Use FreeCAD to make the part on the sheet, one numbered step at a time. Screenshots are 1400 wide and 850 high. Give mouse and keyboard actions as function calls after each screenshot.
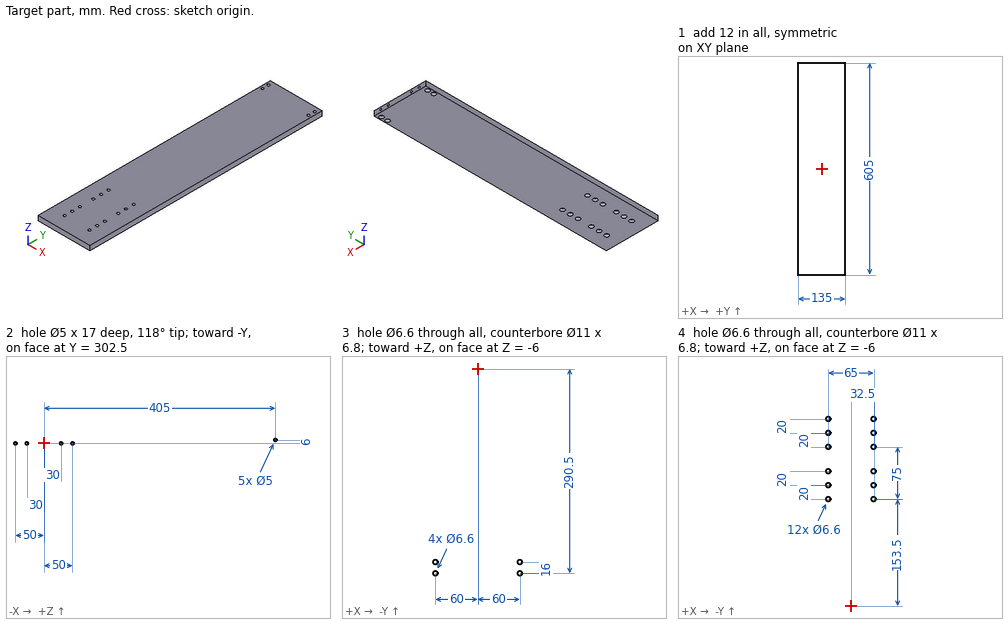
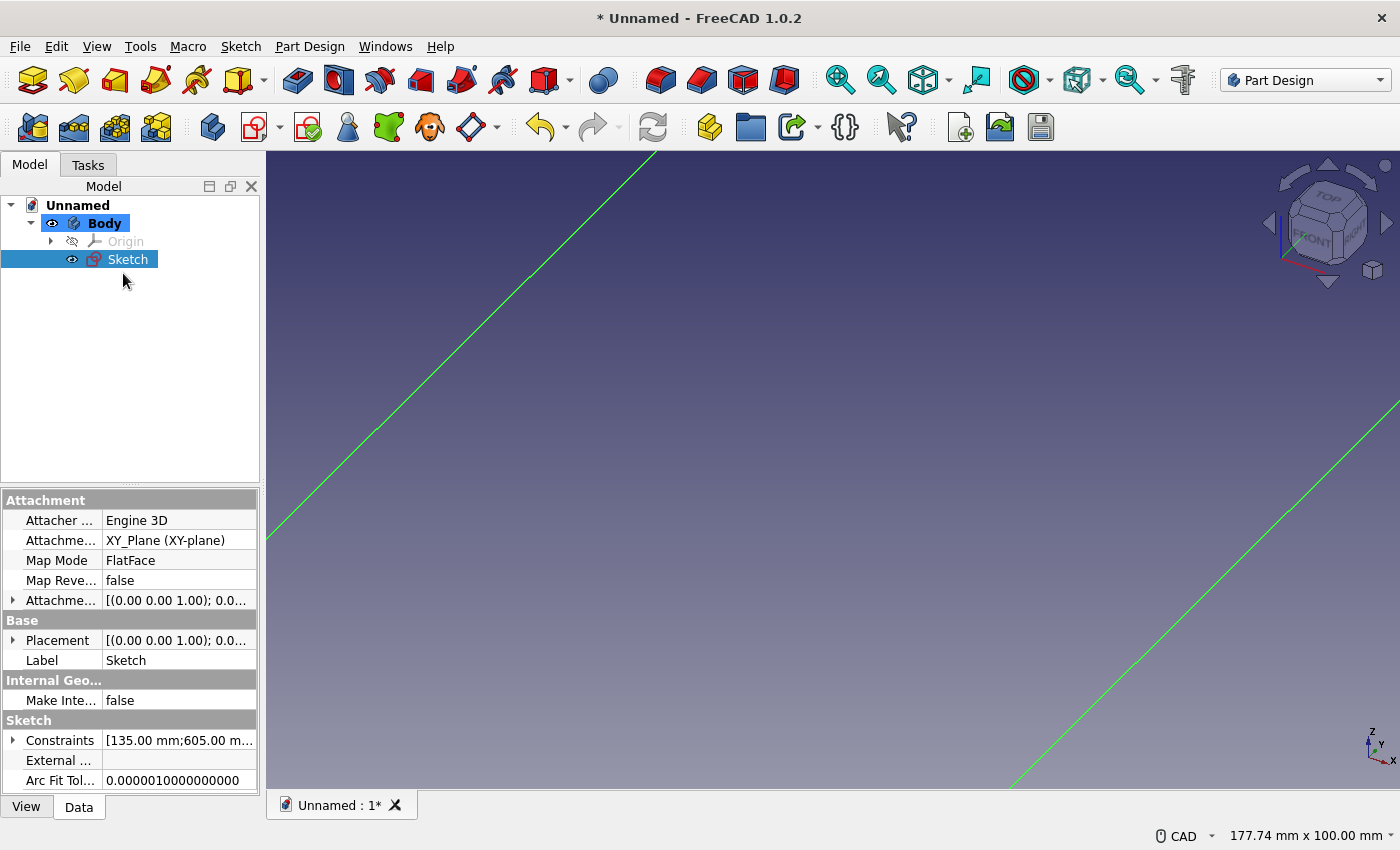
click(33, 80)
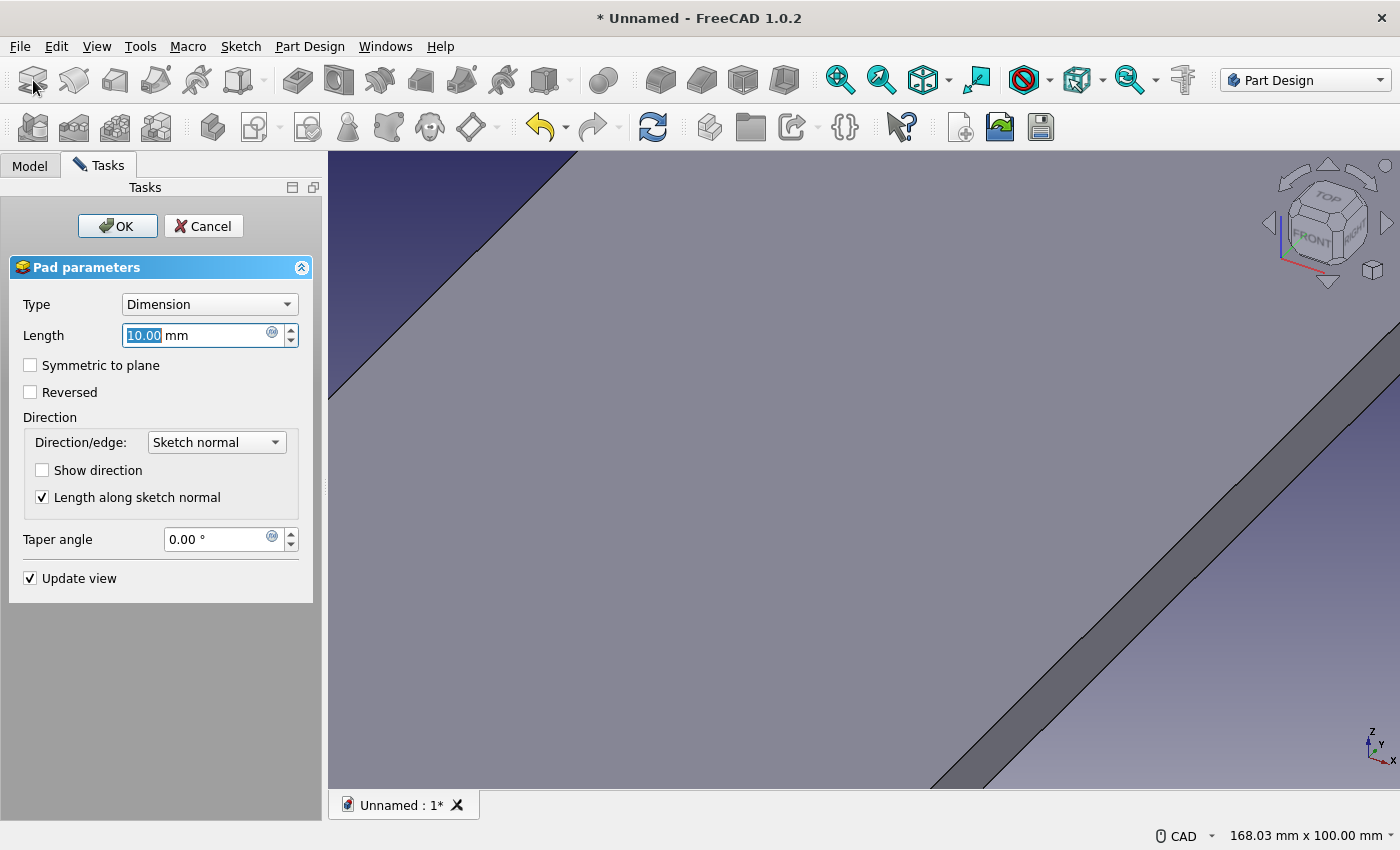
text(12)
key(Tab)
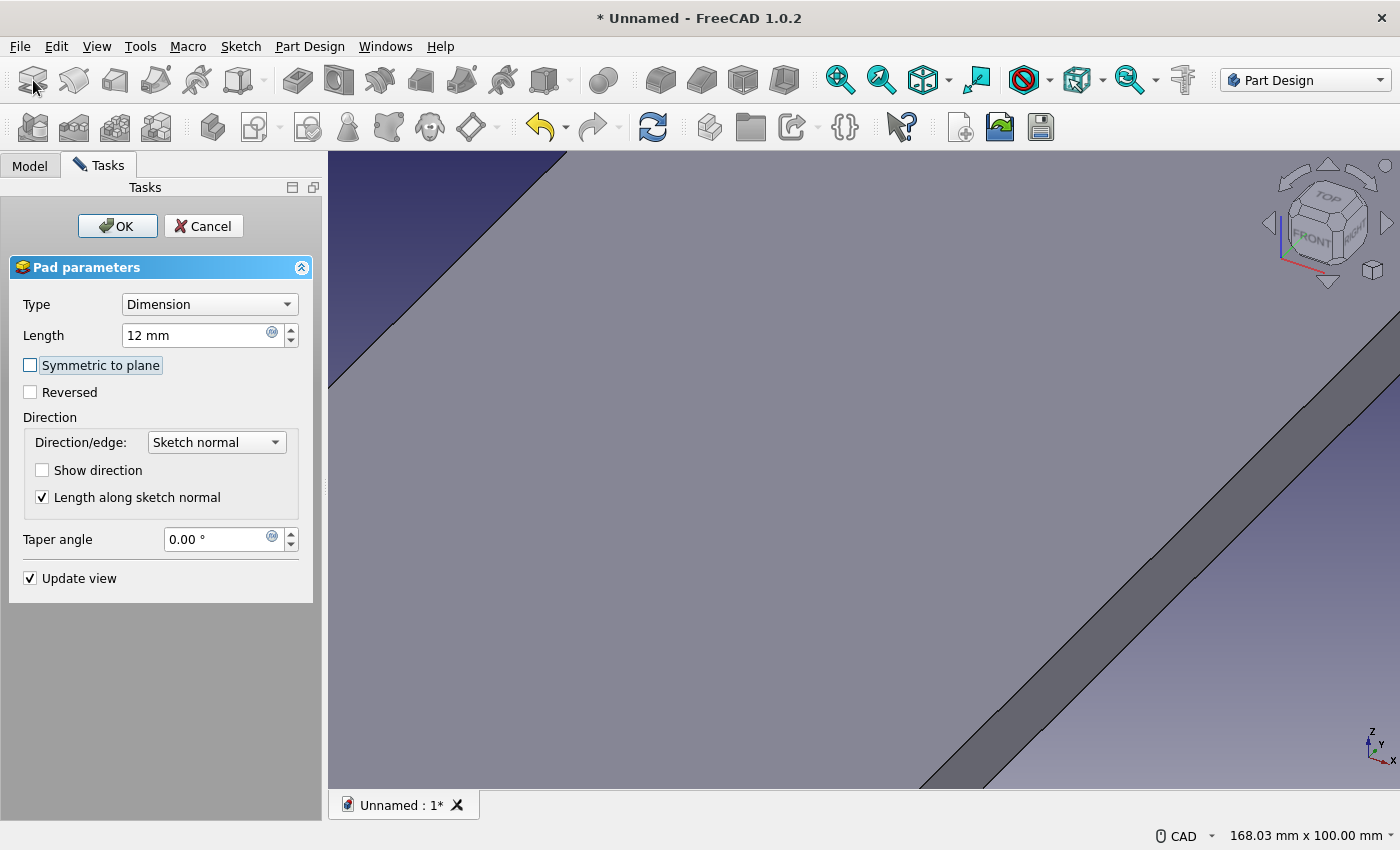
click(31, 365)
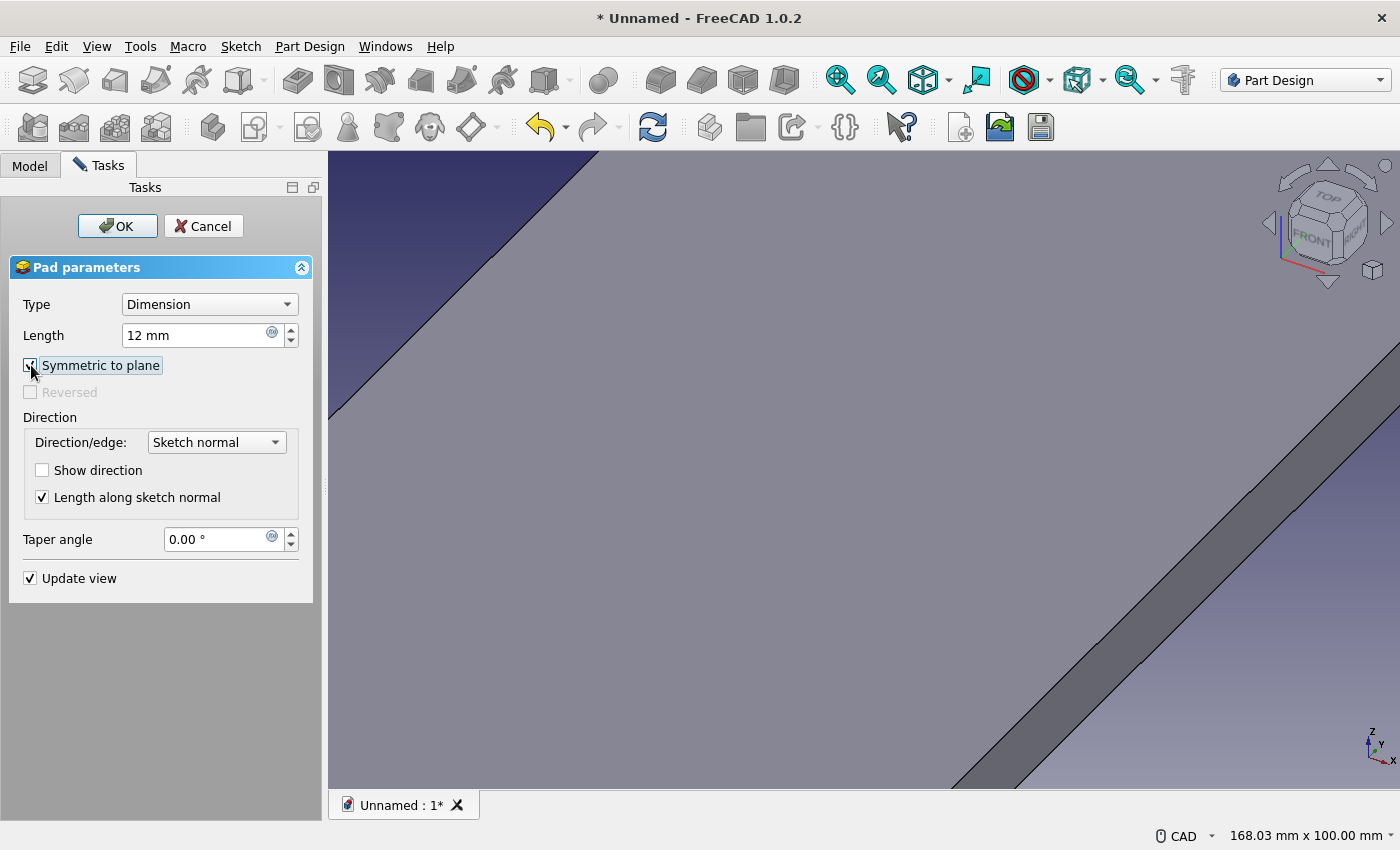
click(118, 226)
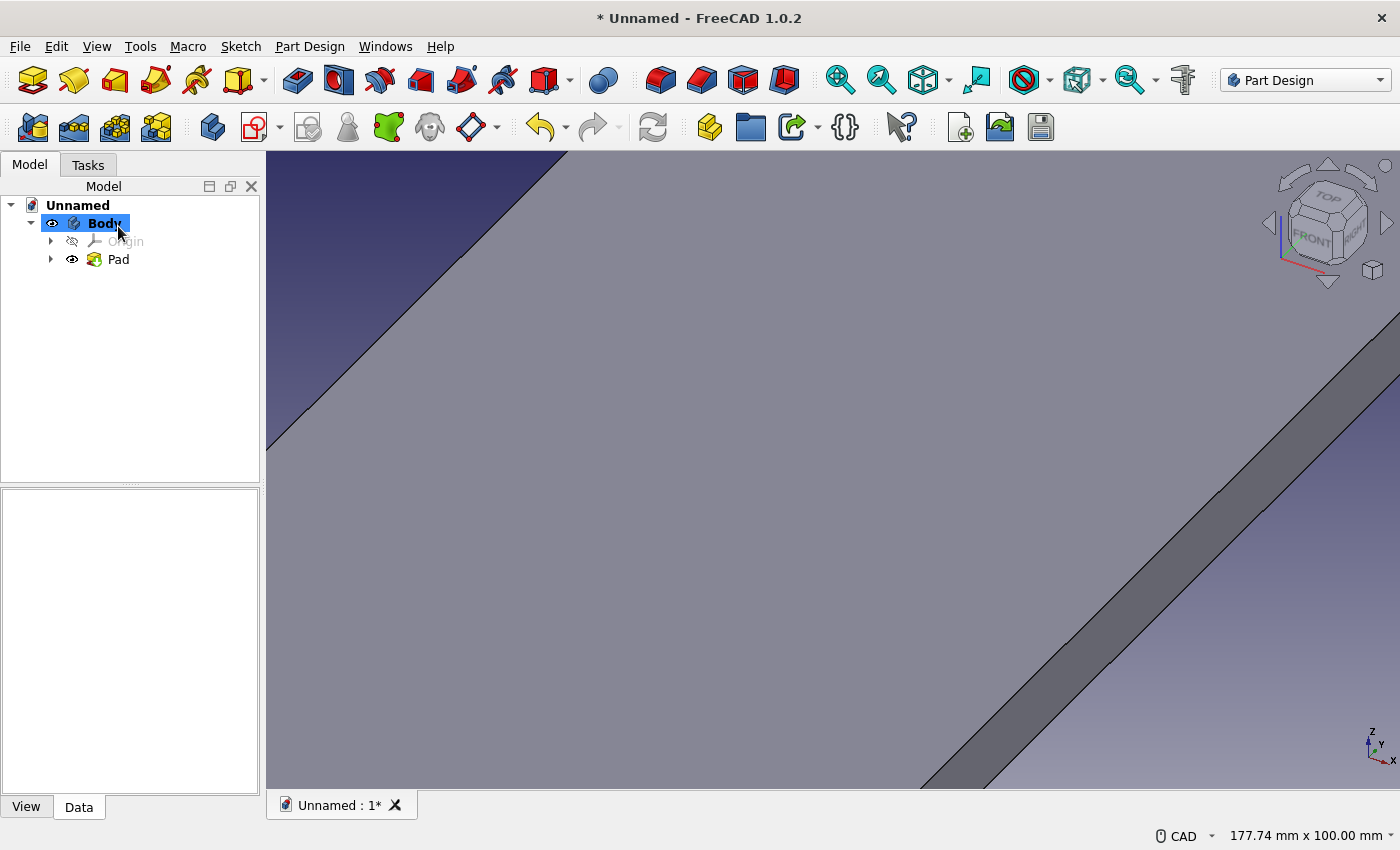
key(v)
key(f)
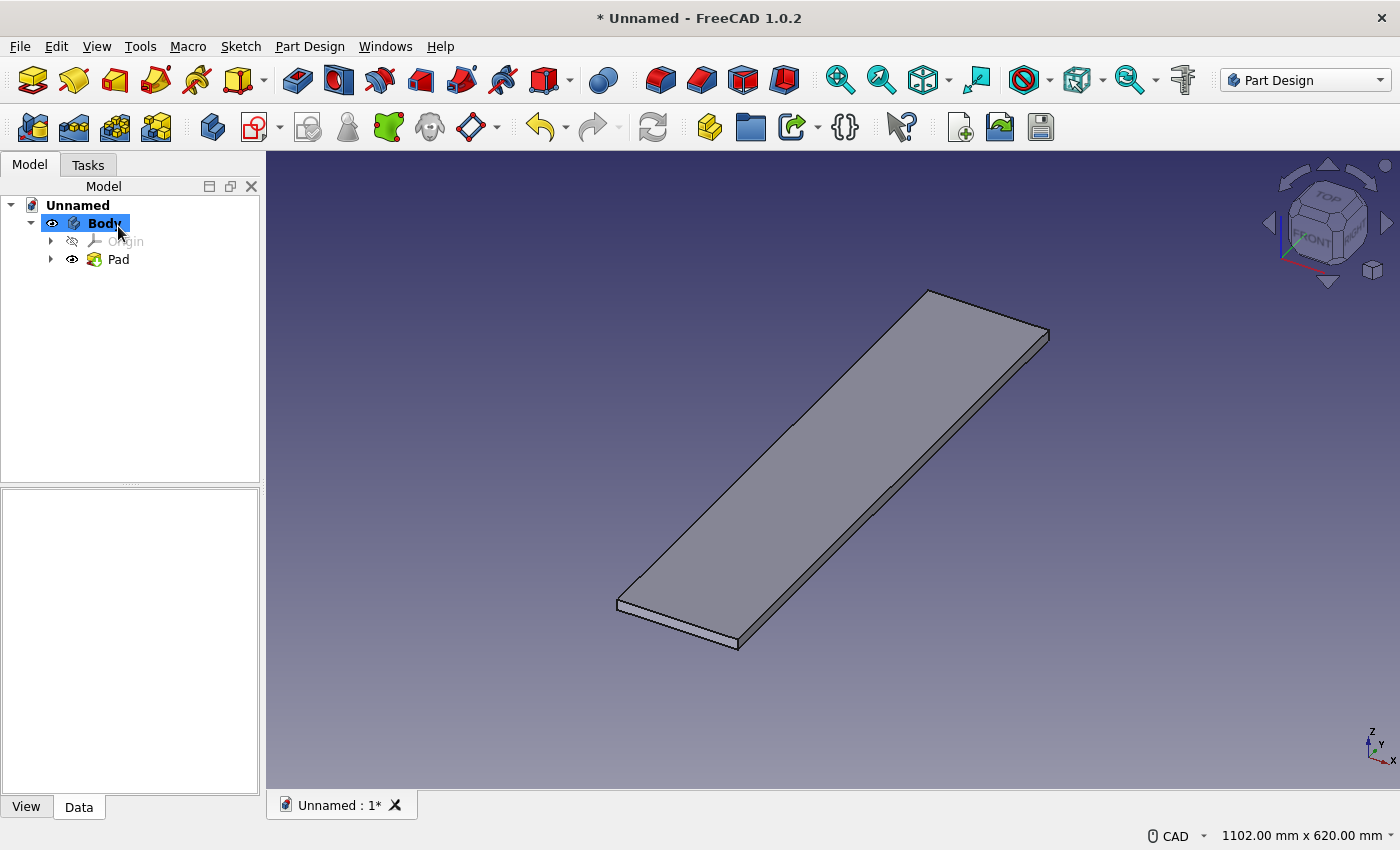
key(4)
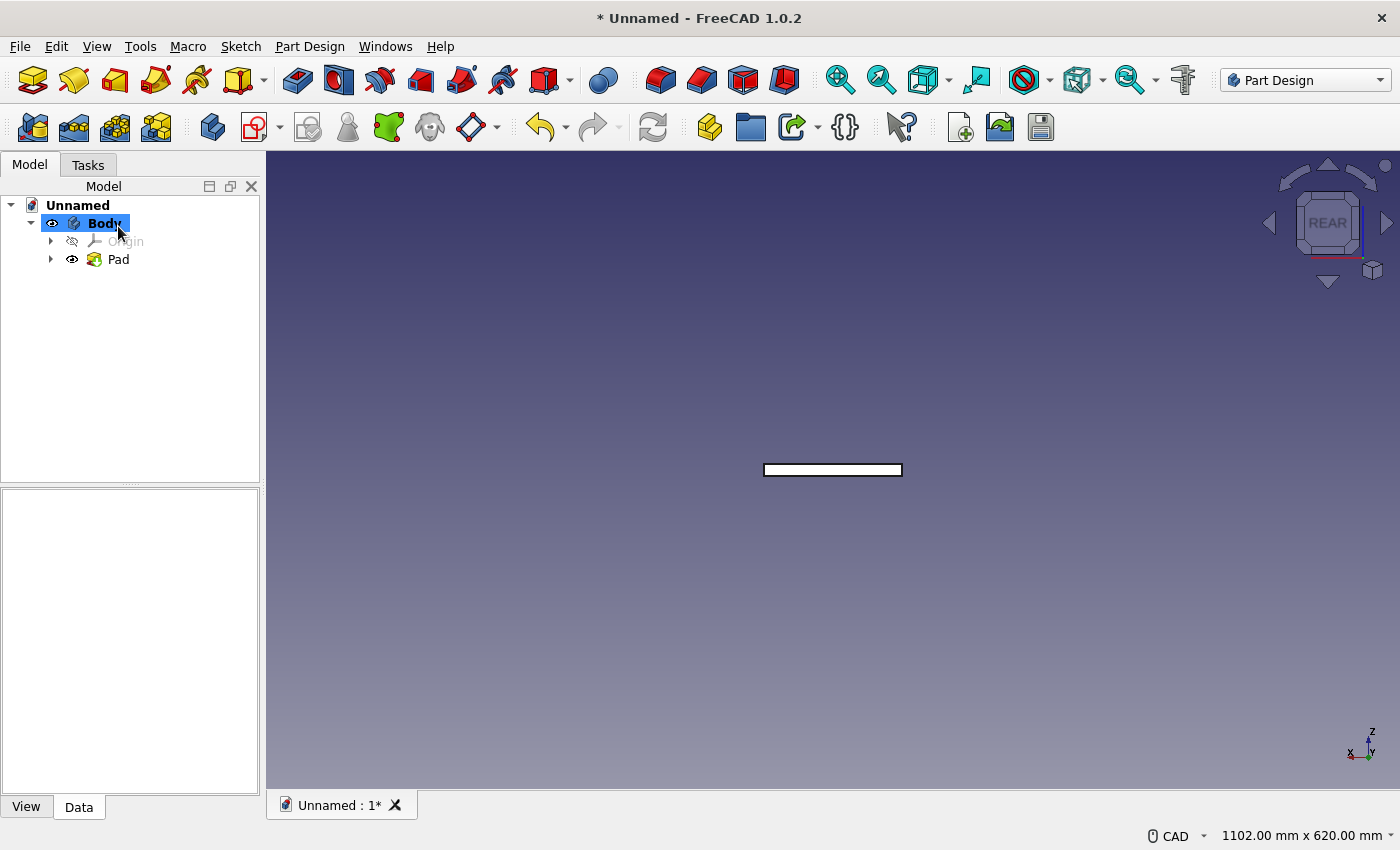
click(841, 80)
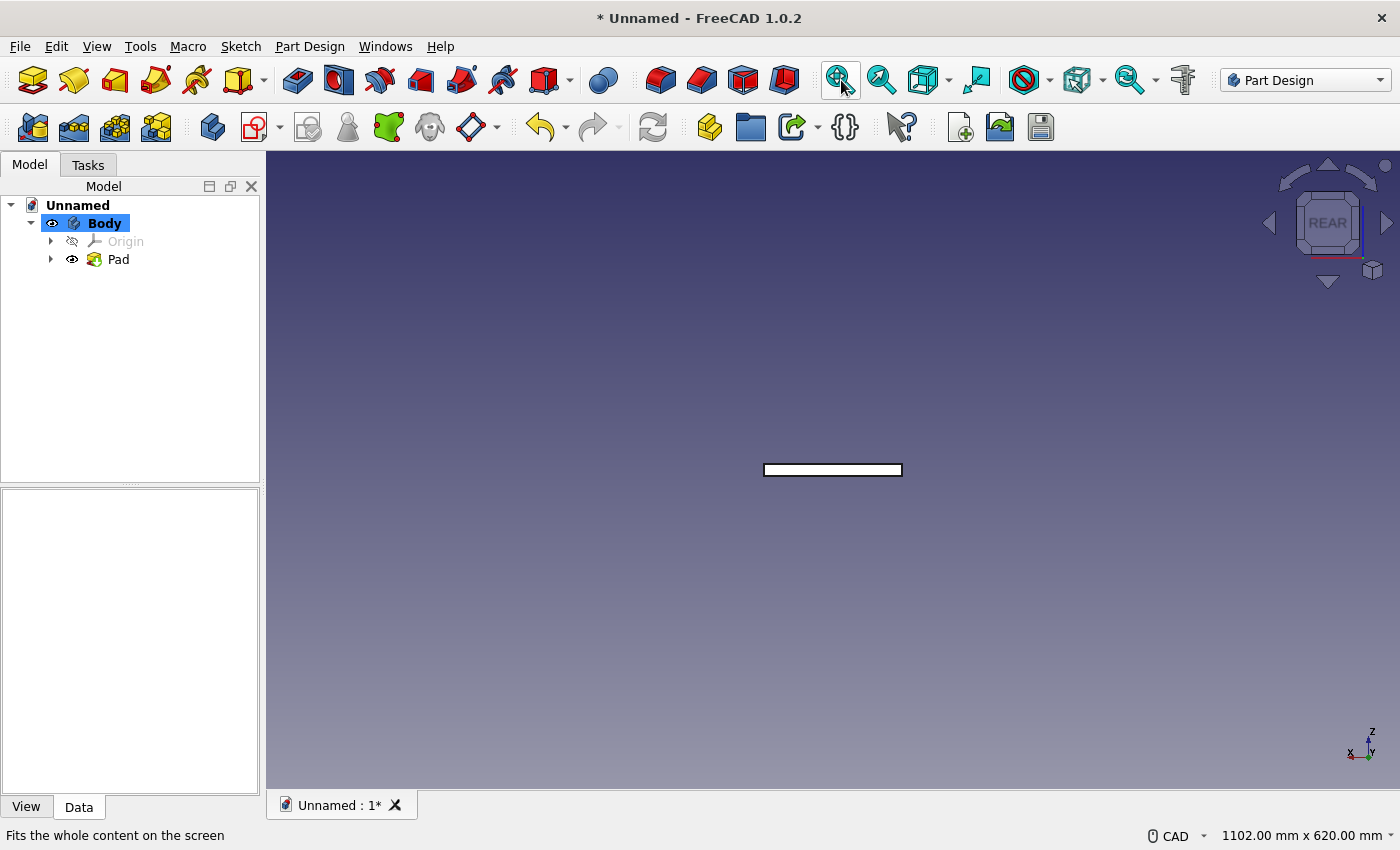
scroll(773, 469, up, 4)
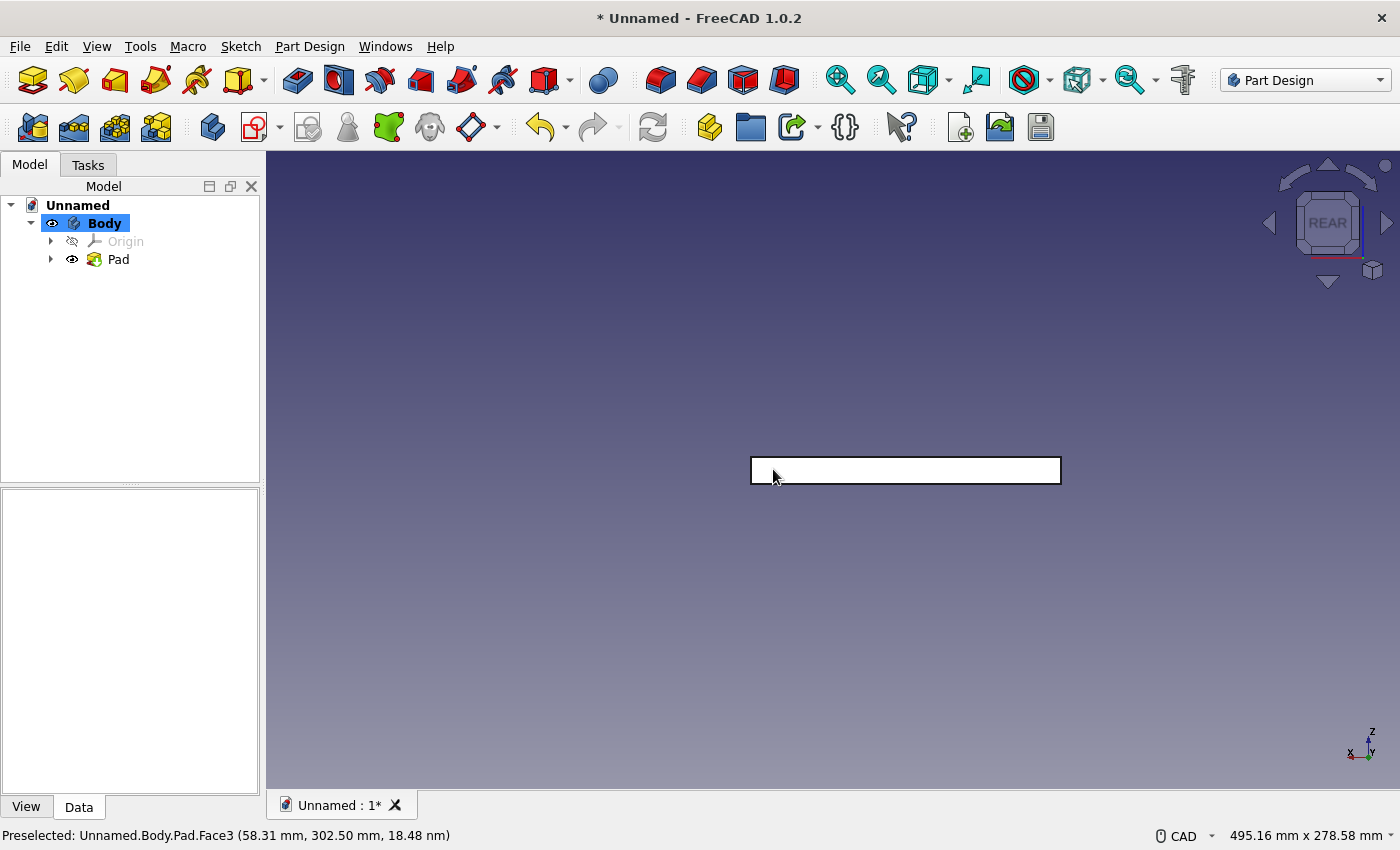
click(773, 470)